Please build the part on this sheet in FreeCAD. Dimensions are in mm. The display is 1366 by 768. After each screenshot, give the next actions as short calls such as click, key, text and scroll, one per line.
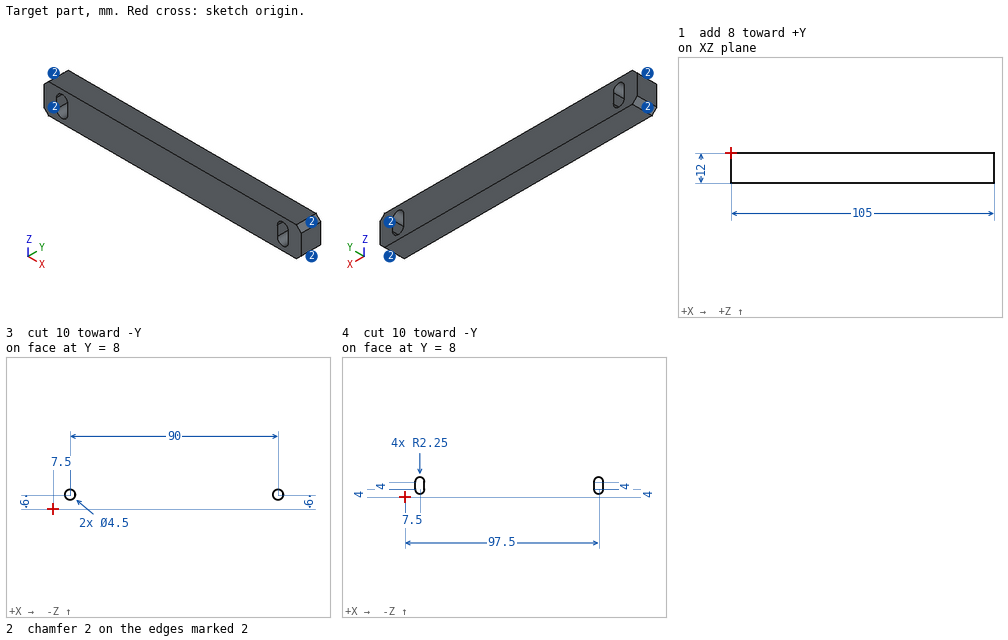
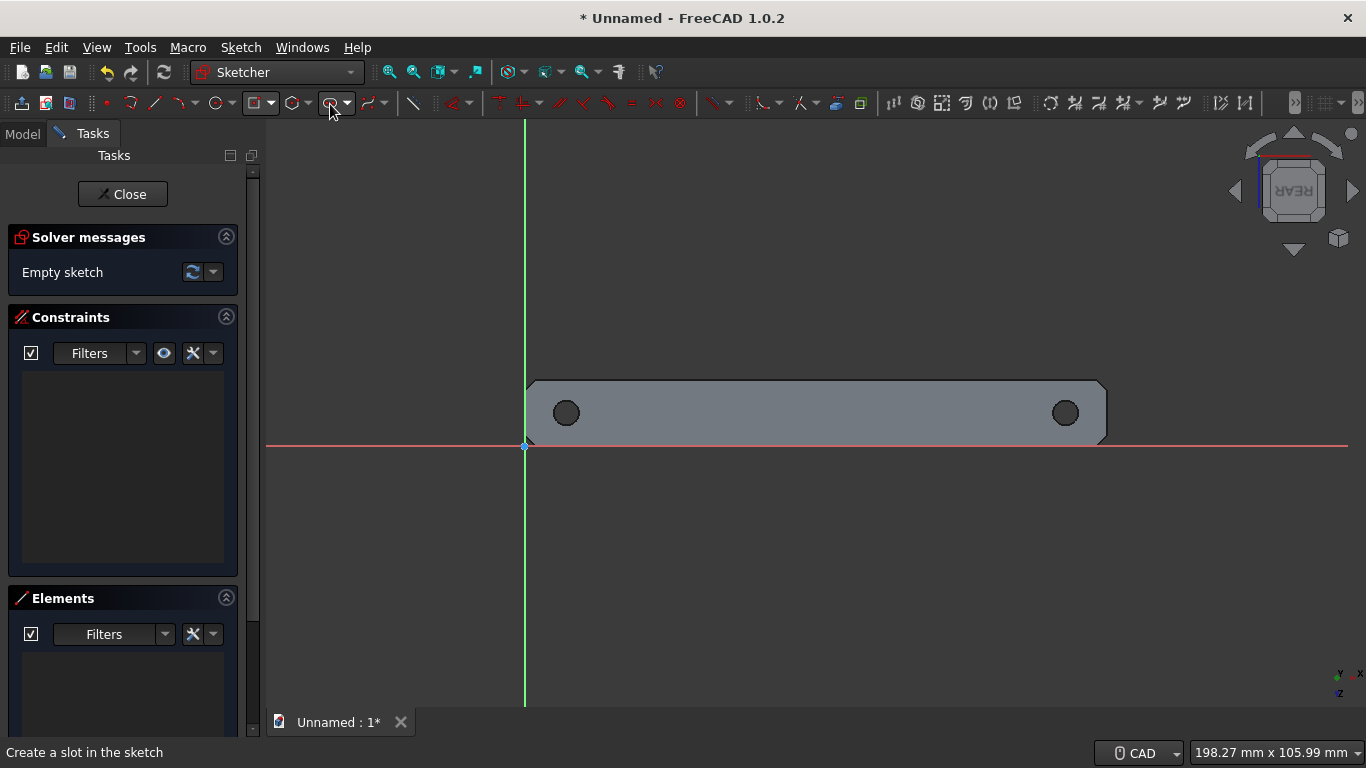
scroll(566, 424, up, 3)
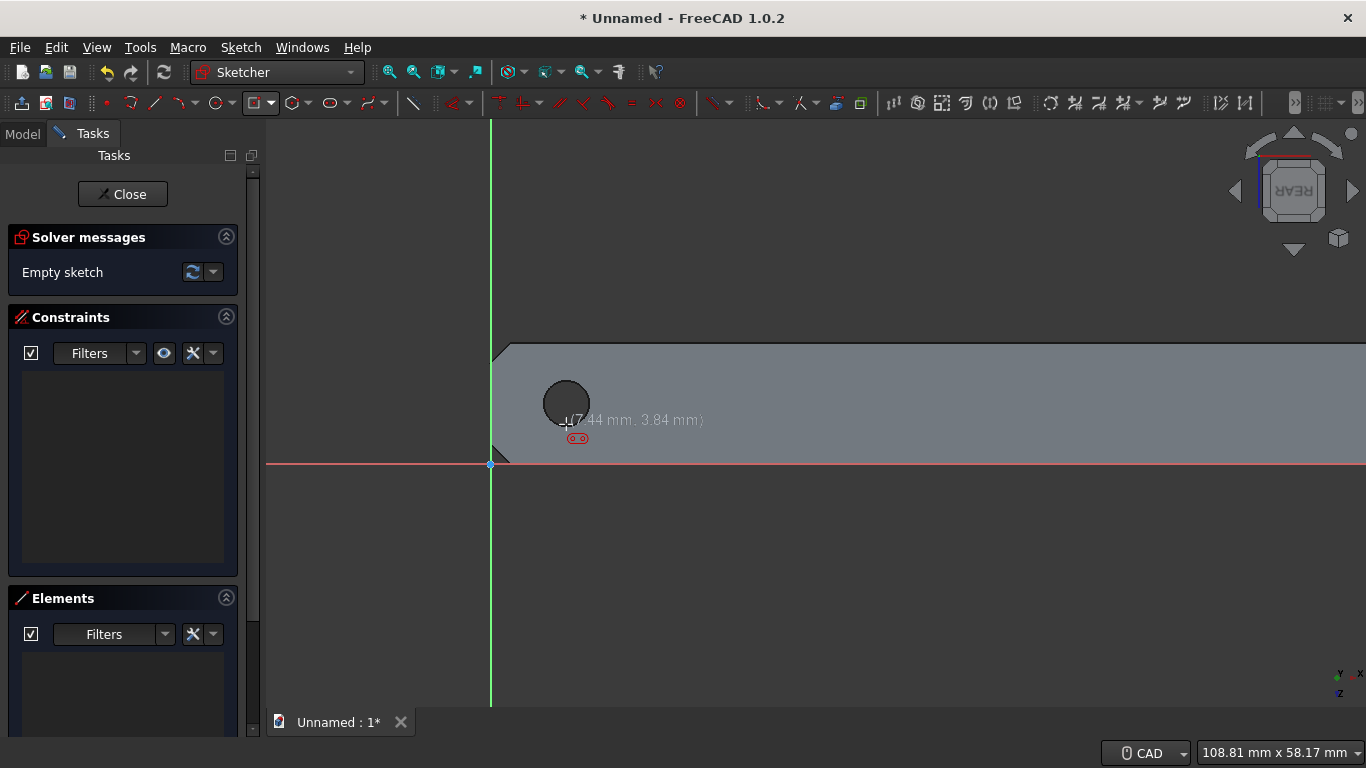
click(566, 424)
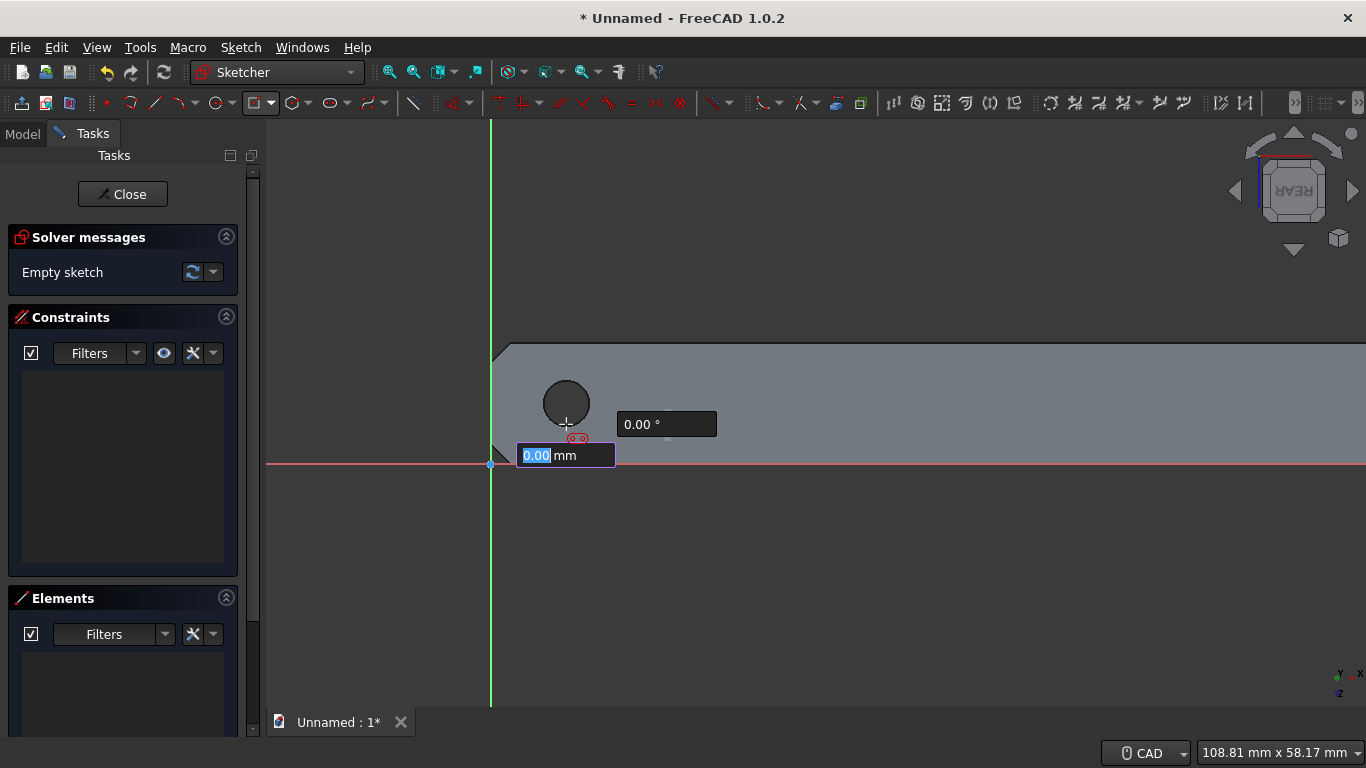
click(566, 383)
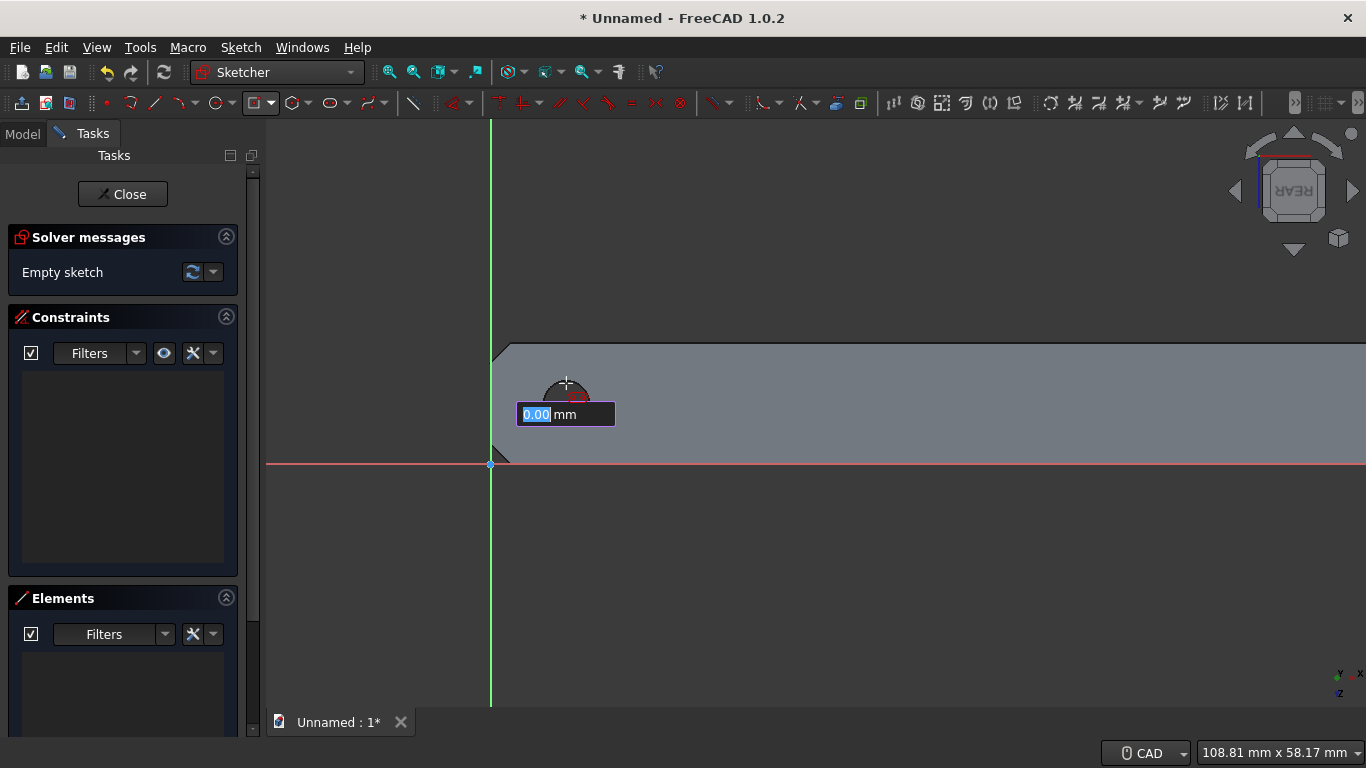
click(544, 404)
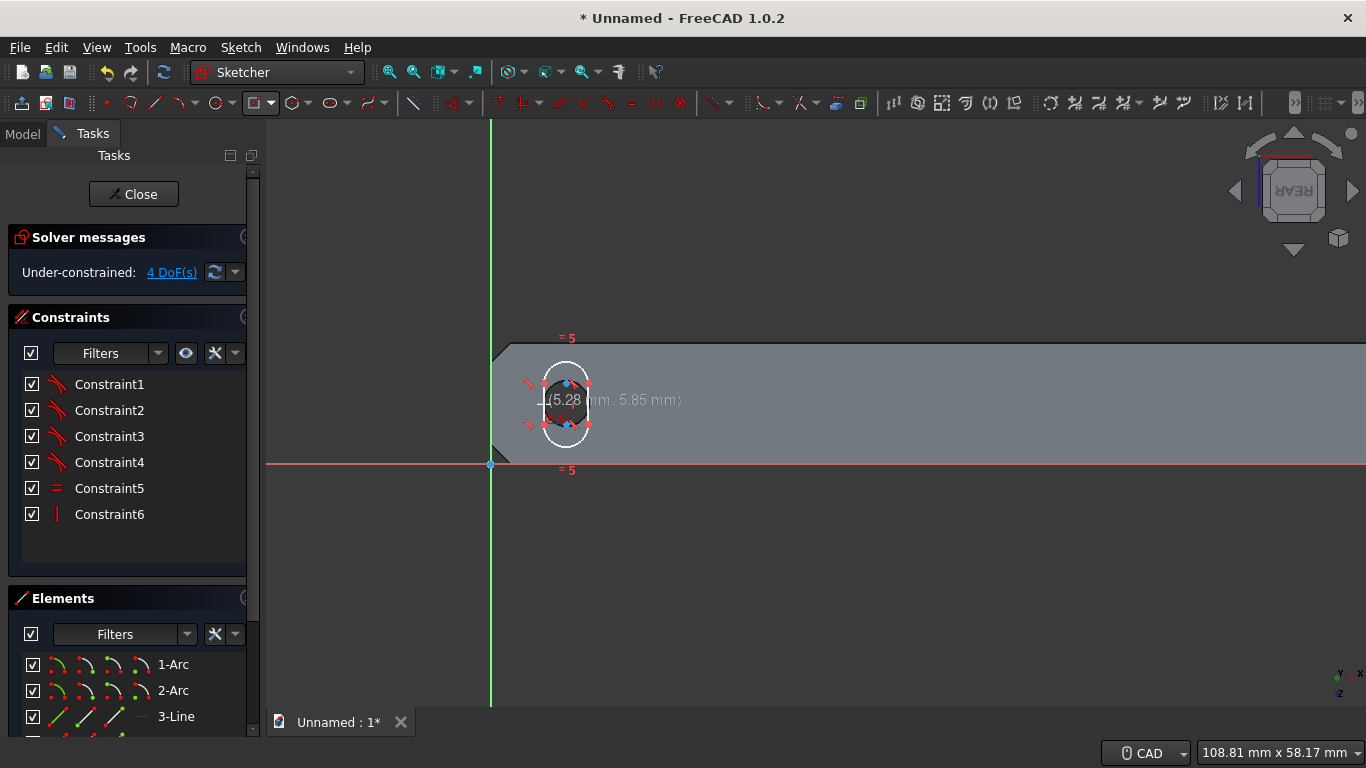
scroll(294, 414, down, 2)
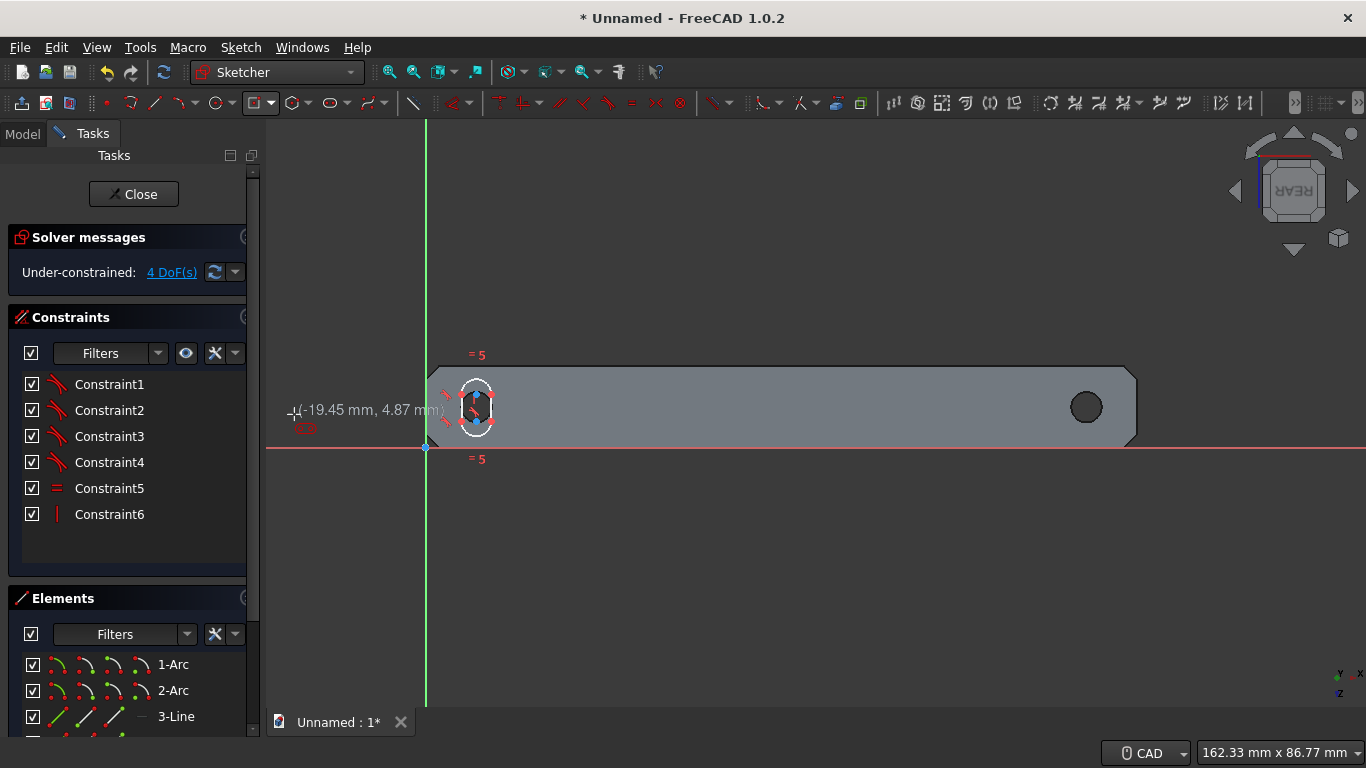
scroll(1086, 421, up, 2)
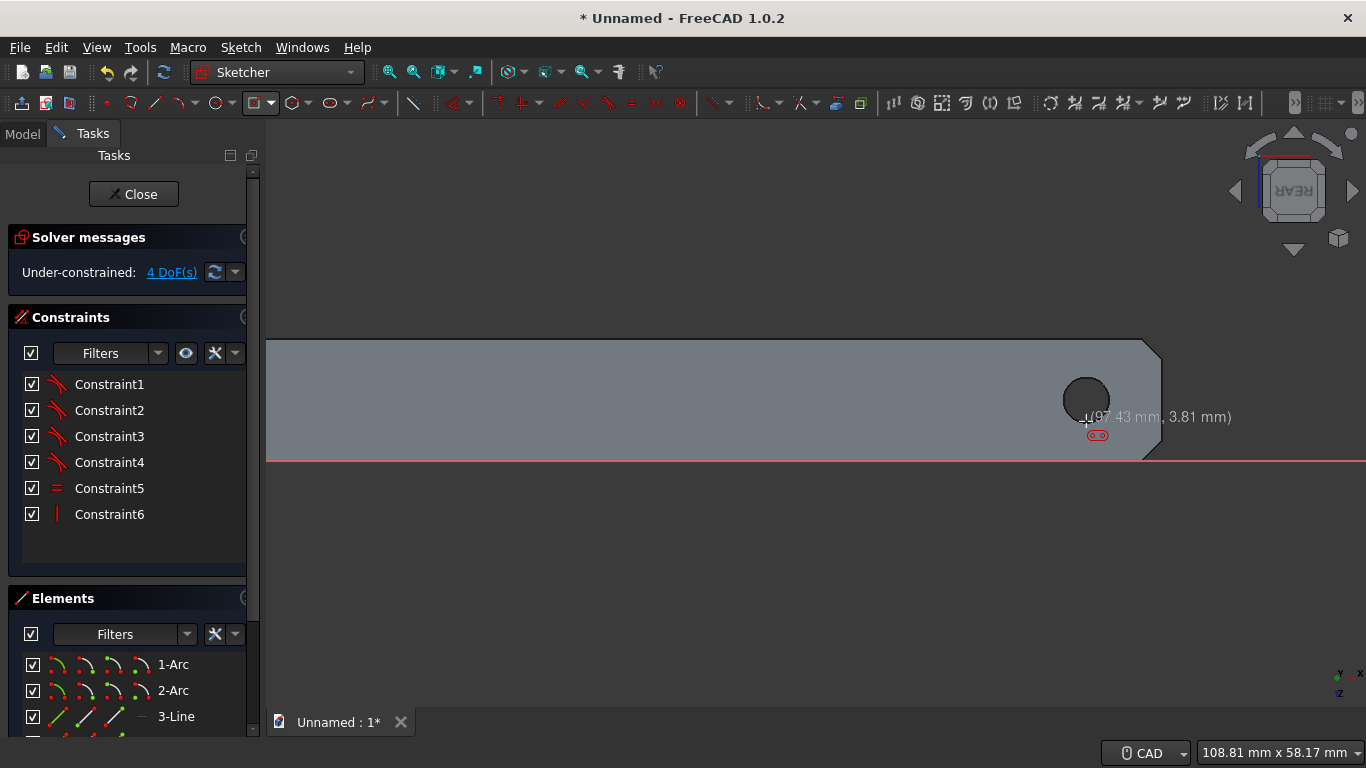
click(1086, 420)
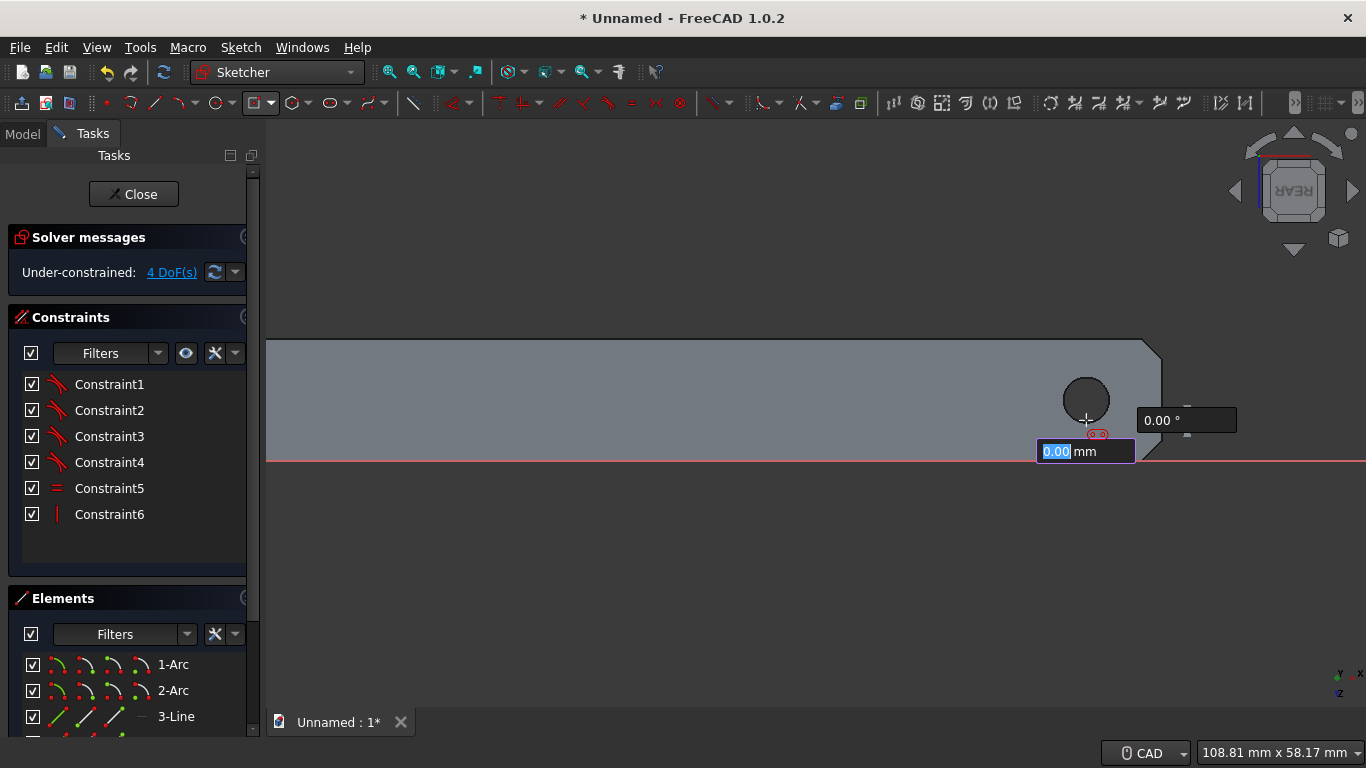
click(1086, 380)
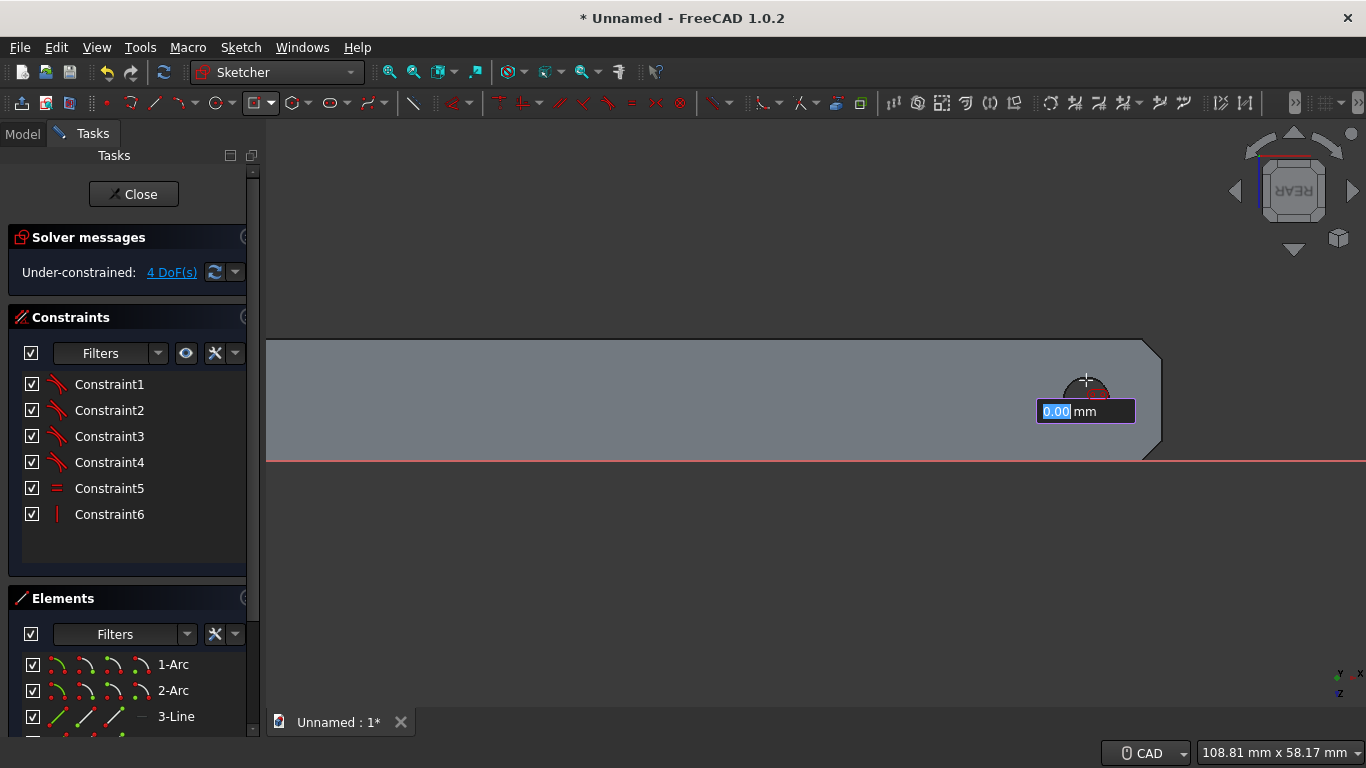
click(1109, 400)
key(Escape)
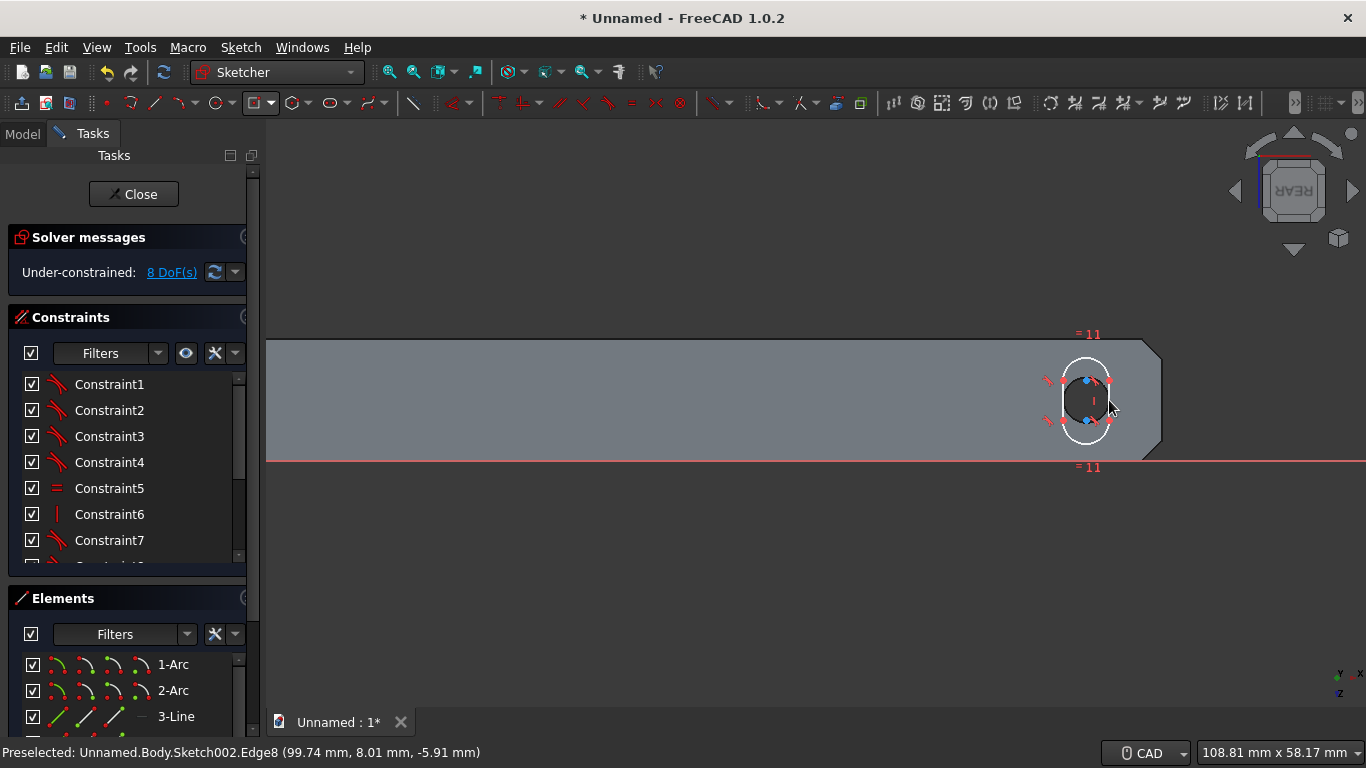
scroll(1037, 421, down, 2)